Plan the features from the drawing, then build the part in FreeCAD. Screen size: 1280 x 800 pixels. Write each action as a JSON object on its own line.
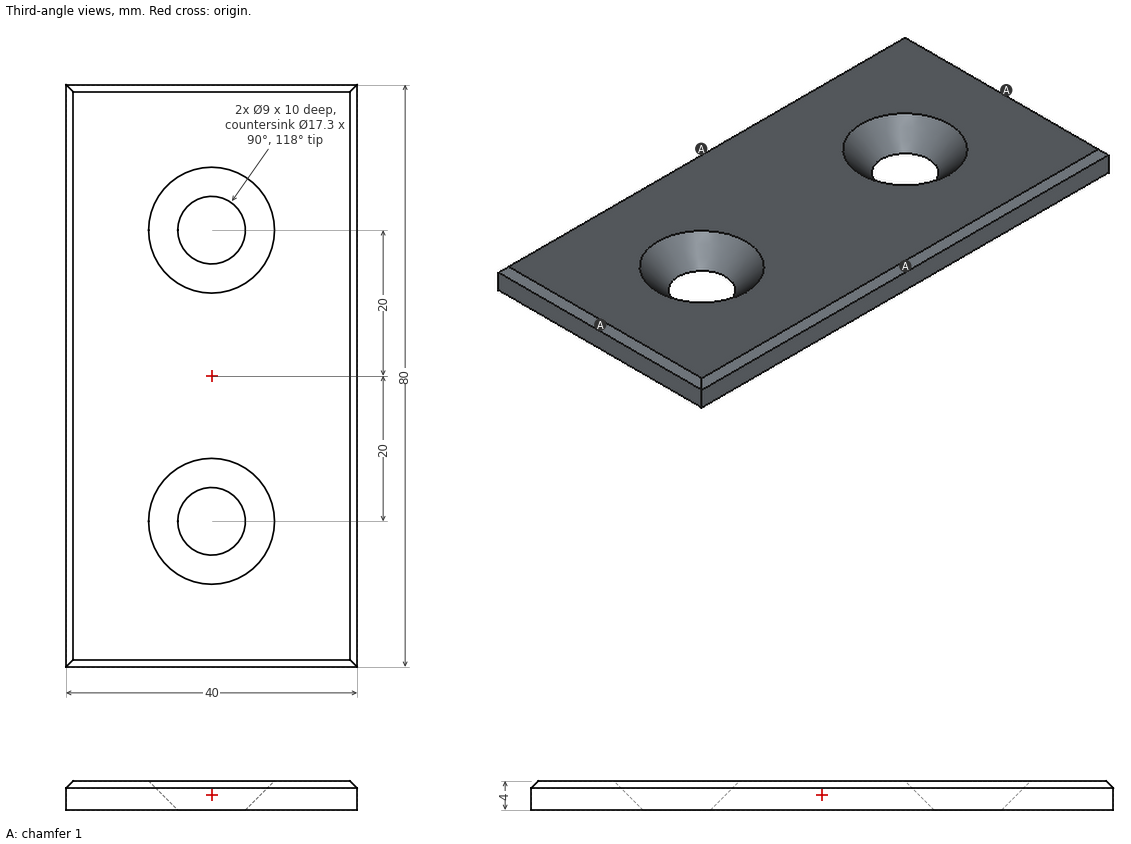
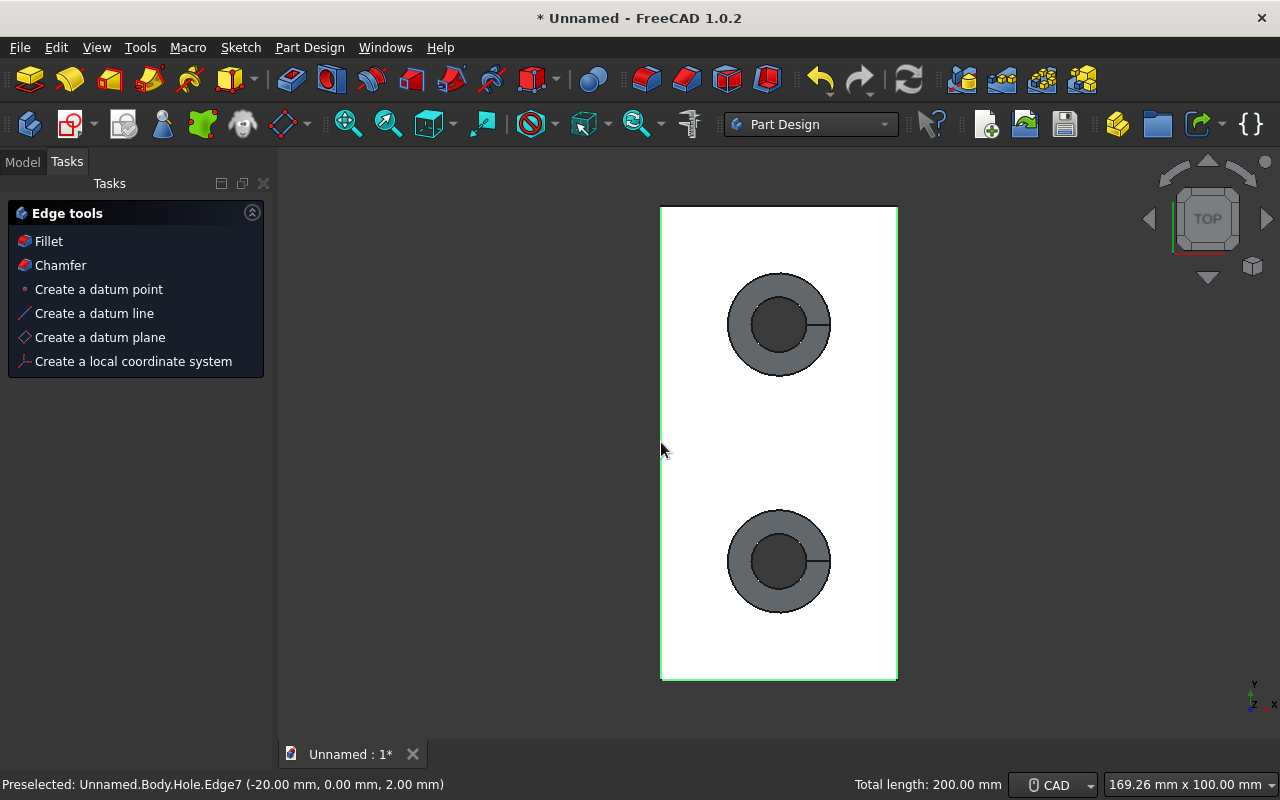
{"action": "left_click", "coordinate": [779, 205], "text": "ctrl"}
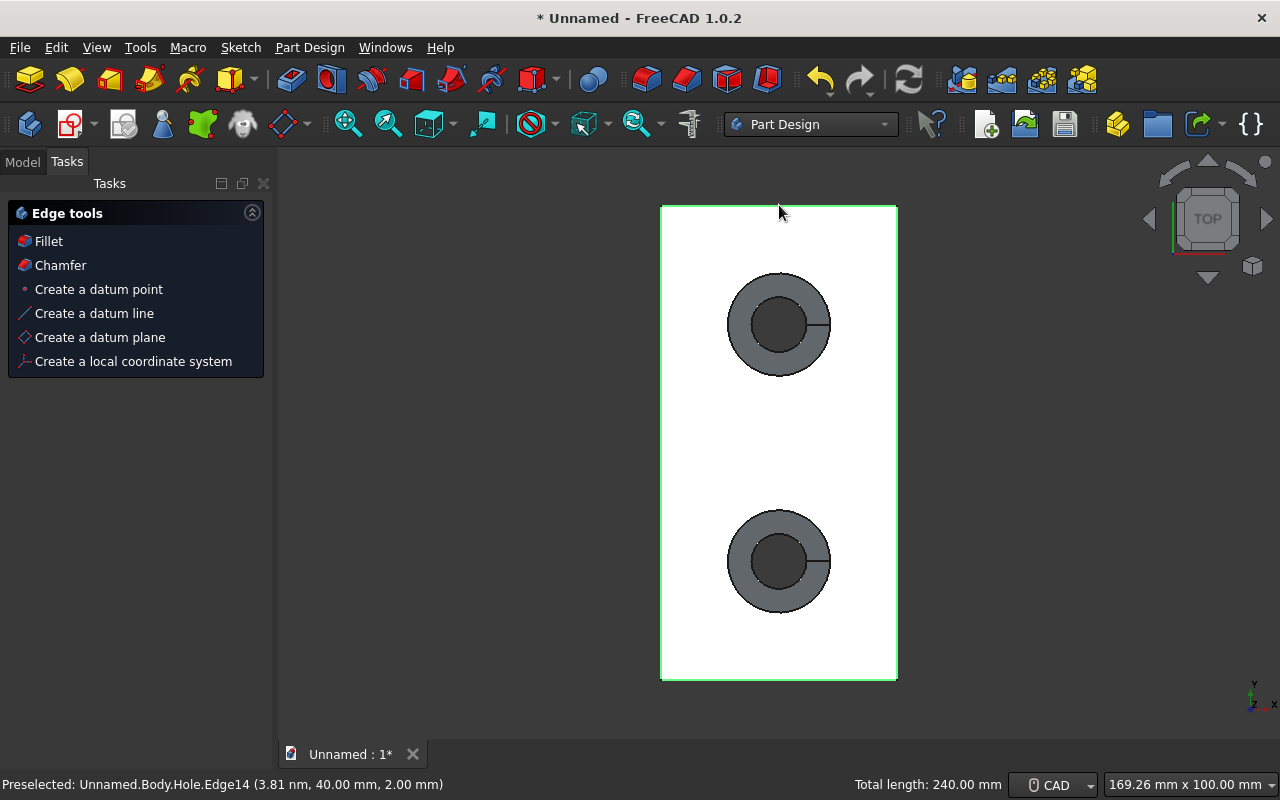
{"action": "left_click", "coordinate": [688, 80]}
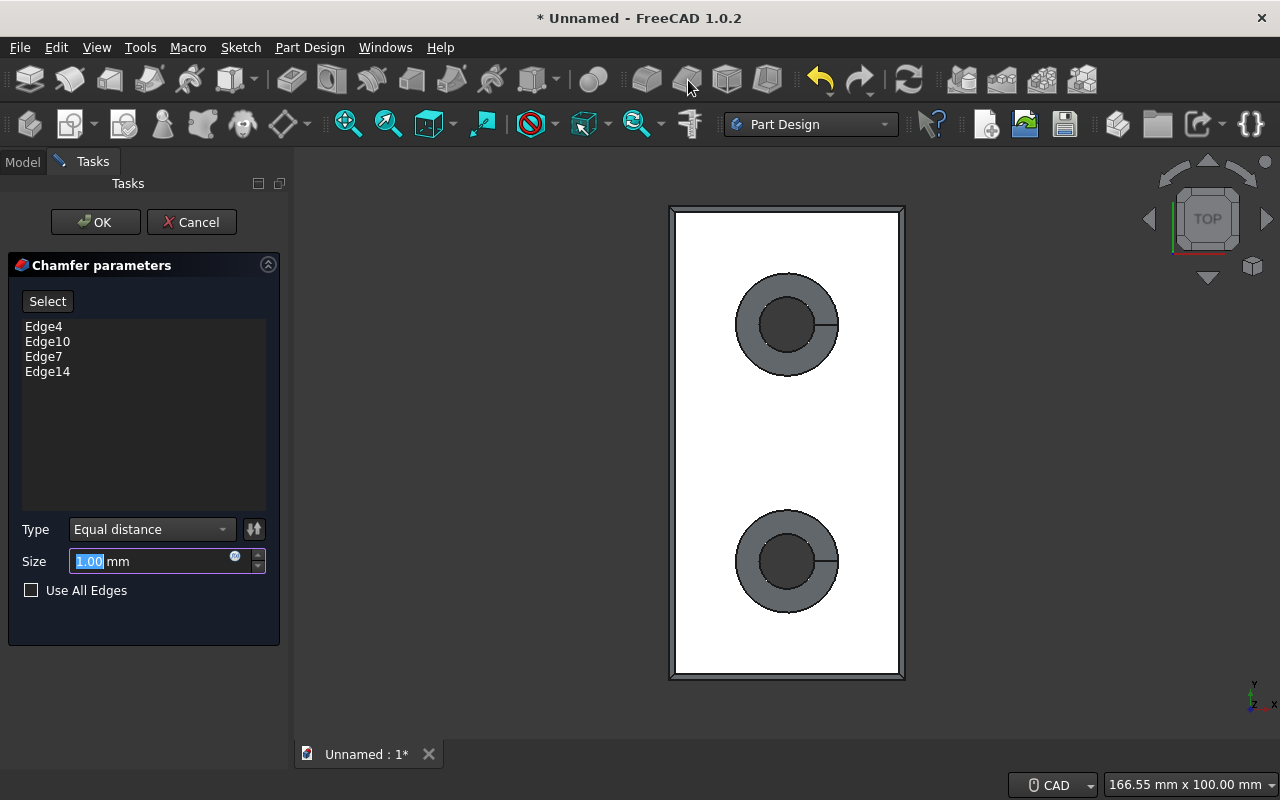
{"action": "type", "text": "1"}
{"action": "key", "text": "Tab"}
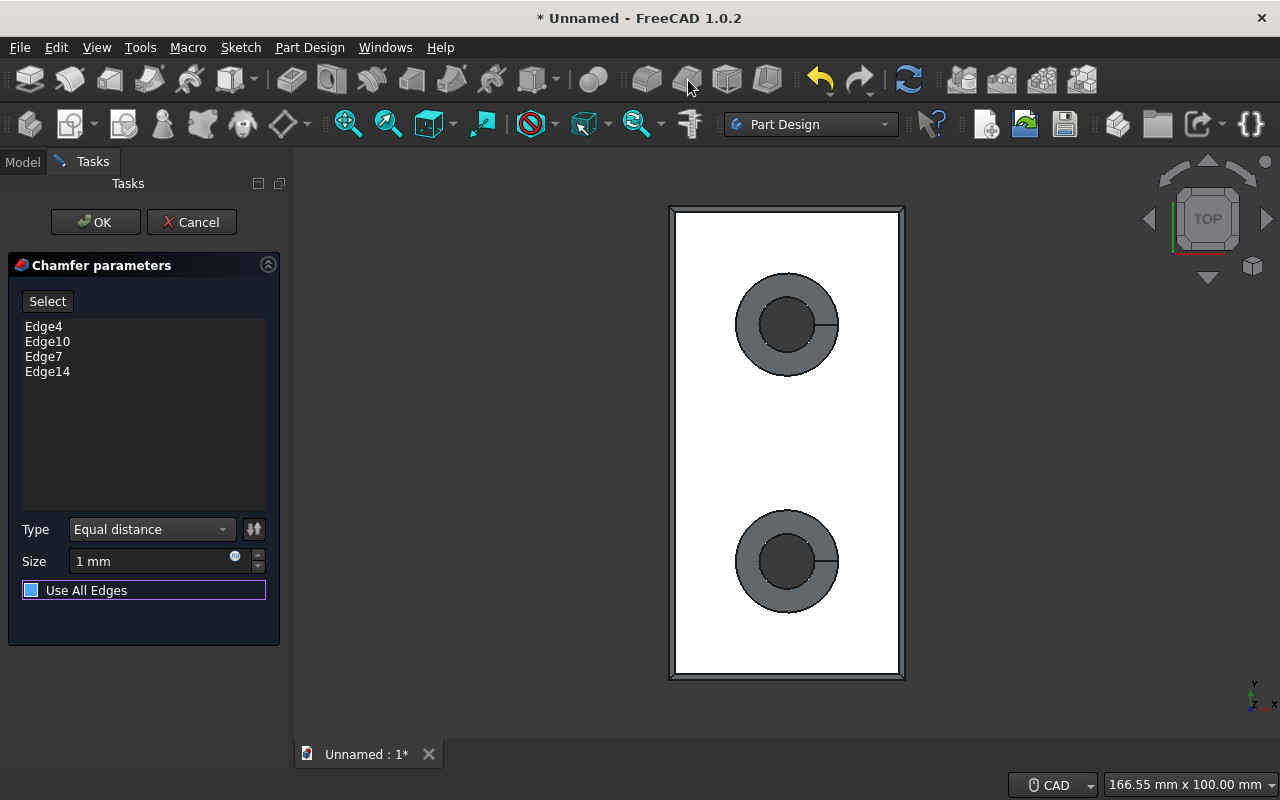
{"action": "left_click", "coordinate": [96, 222]}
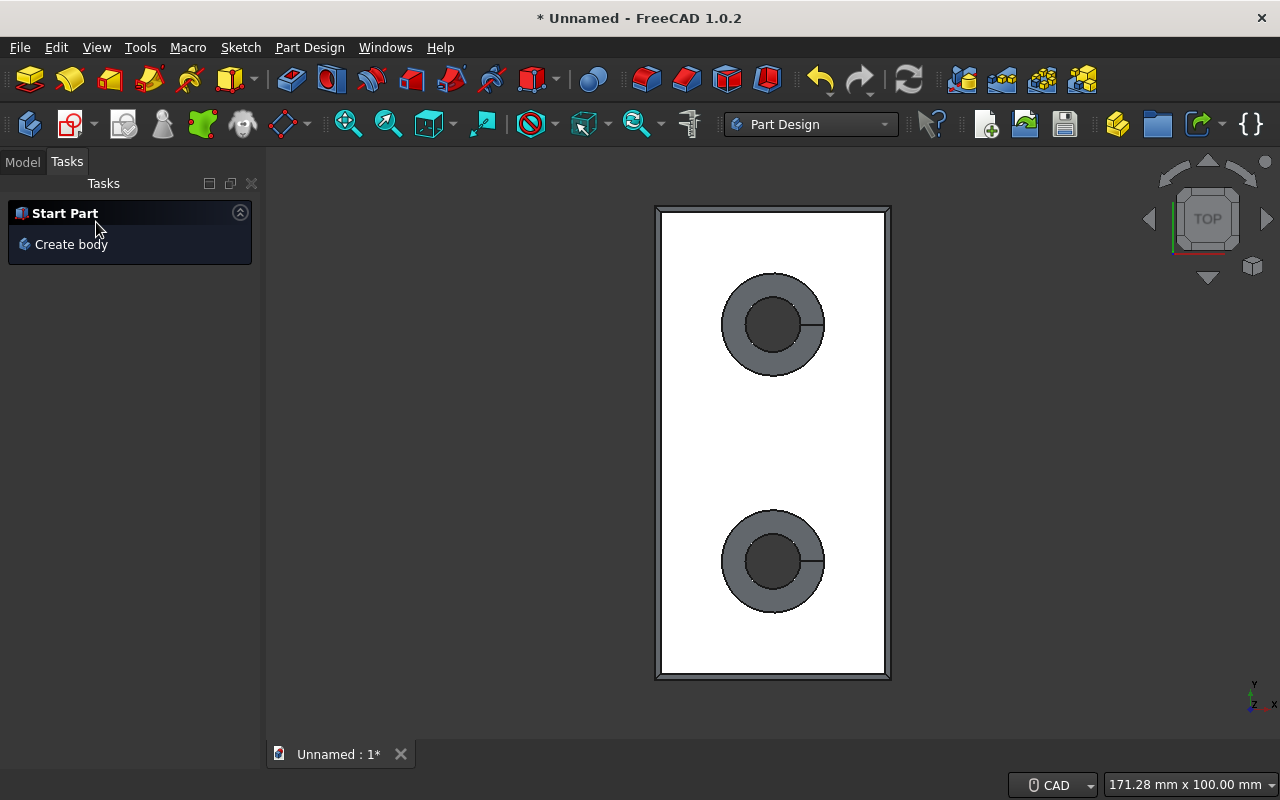
{"action": "key", "text": "0"}